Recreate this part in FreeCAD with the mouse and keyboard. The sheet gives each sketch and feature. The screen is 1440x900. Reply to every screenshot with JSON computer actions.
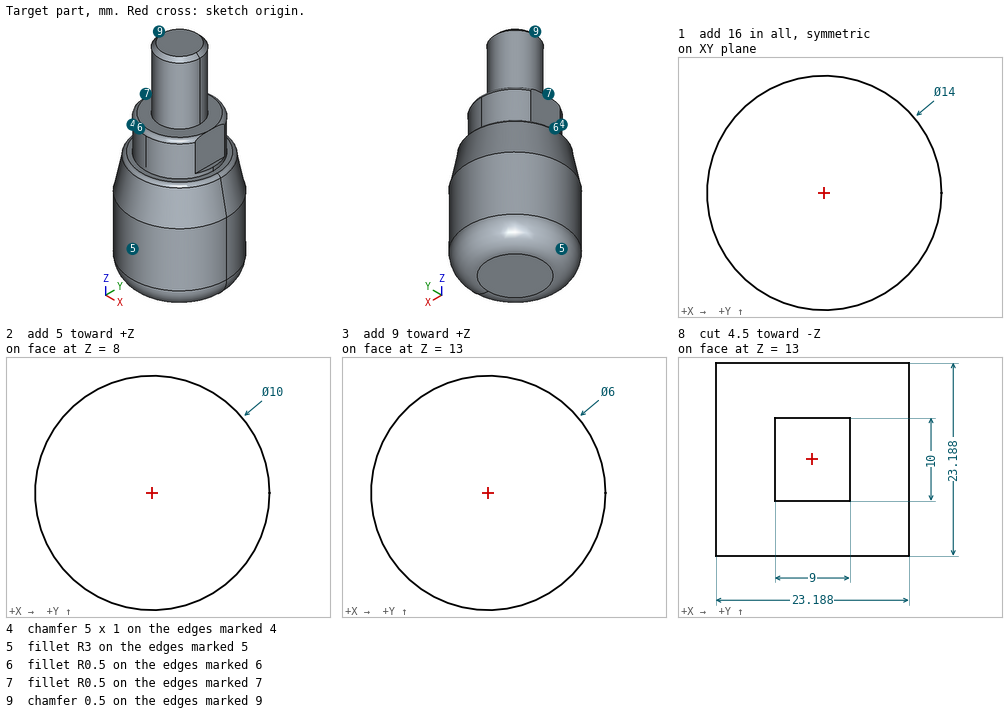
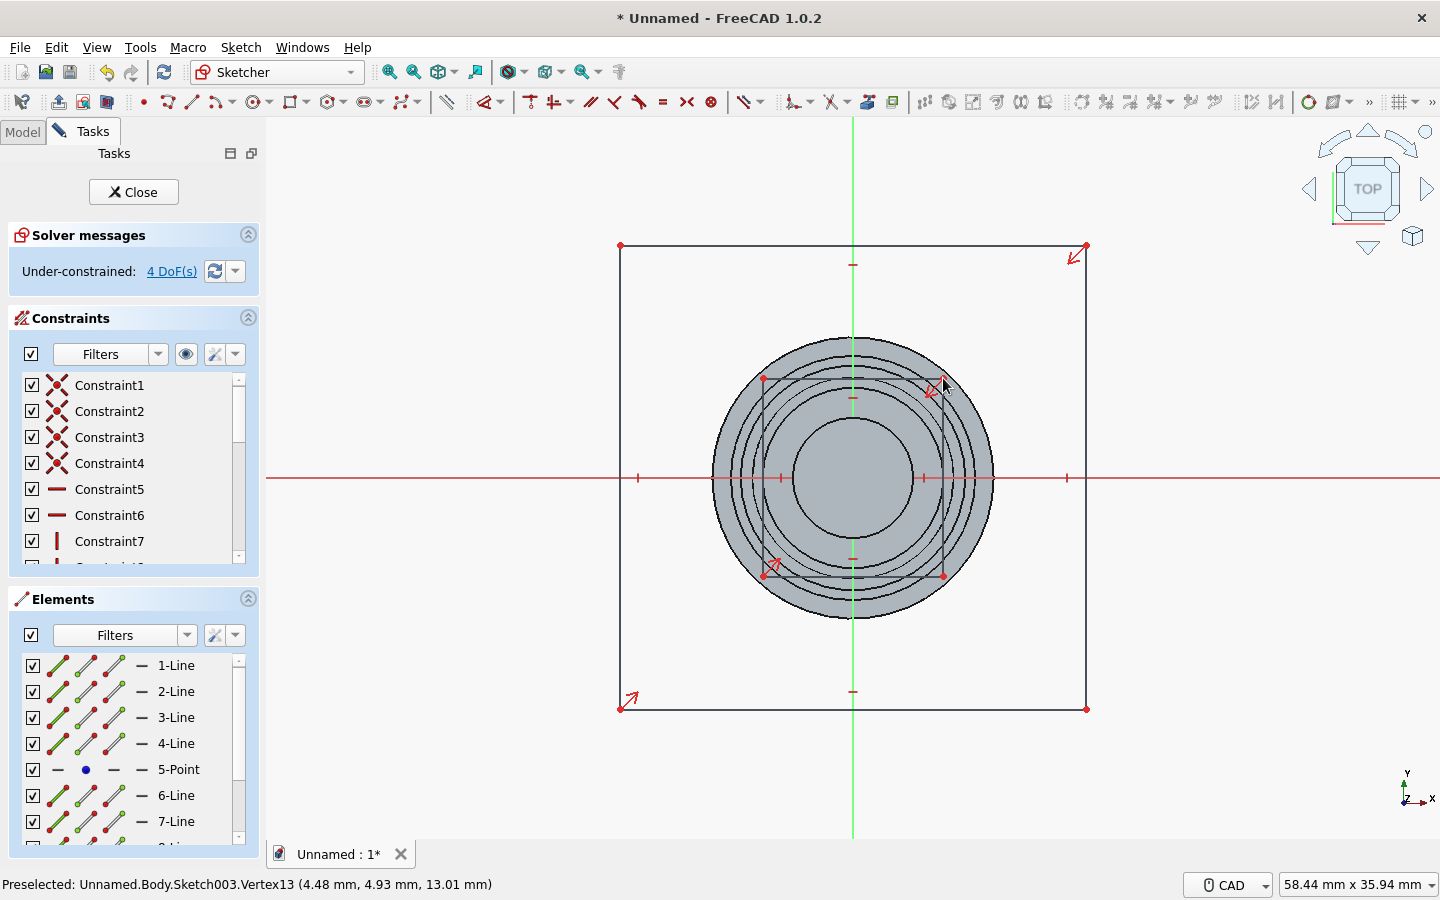
{"action": "left_click", "coordinate": [817, 577]}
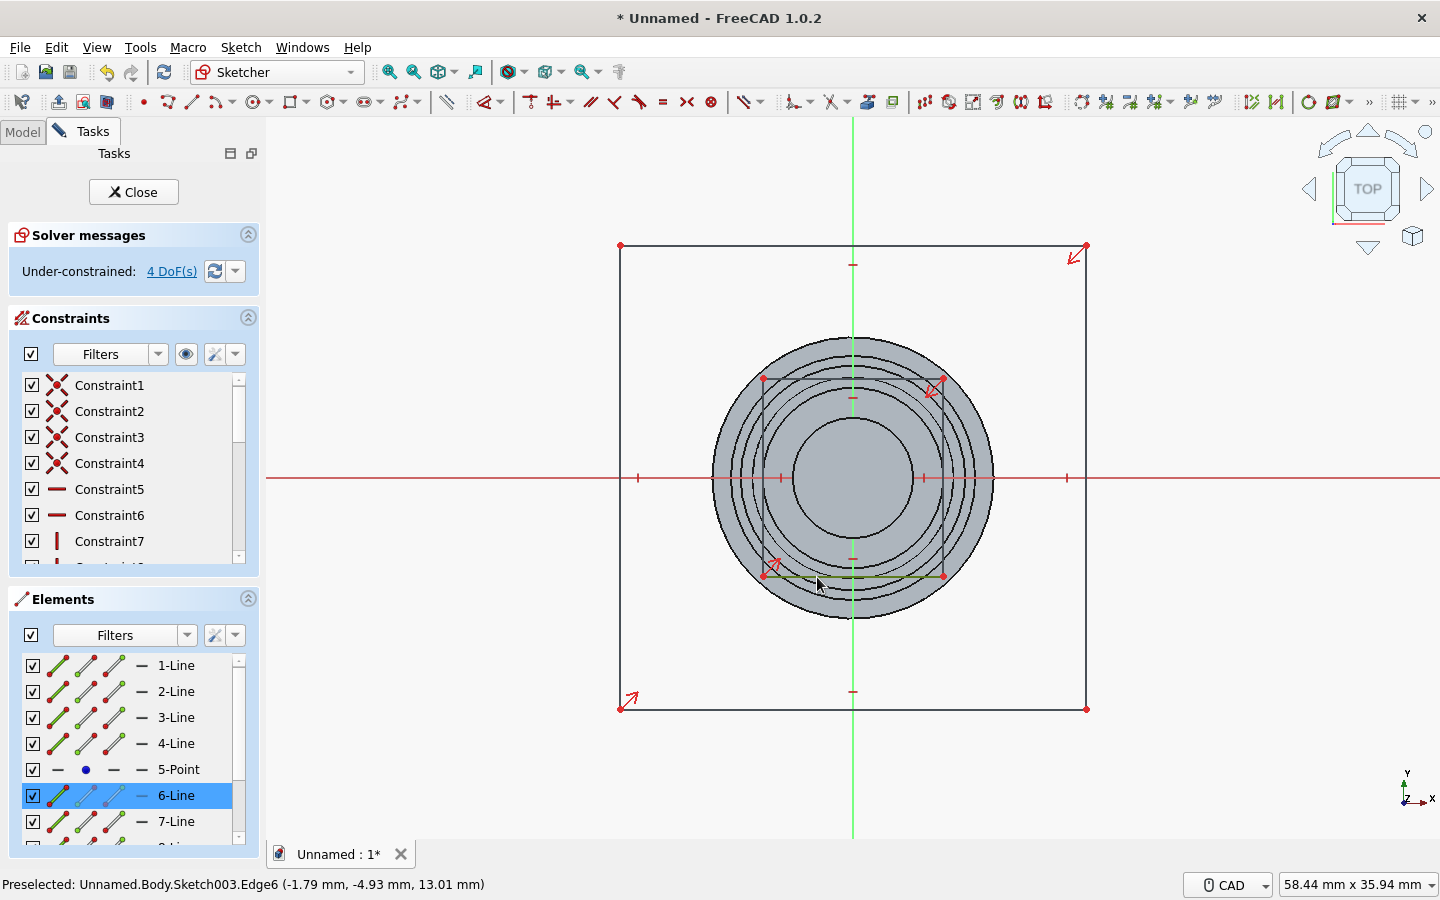
{"action": "key", "text": "l"}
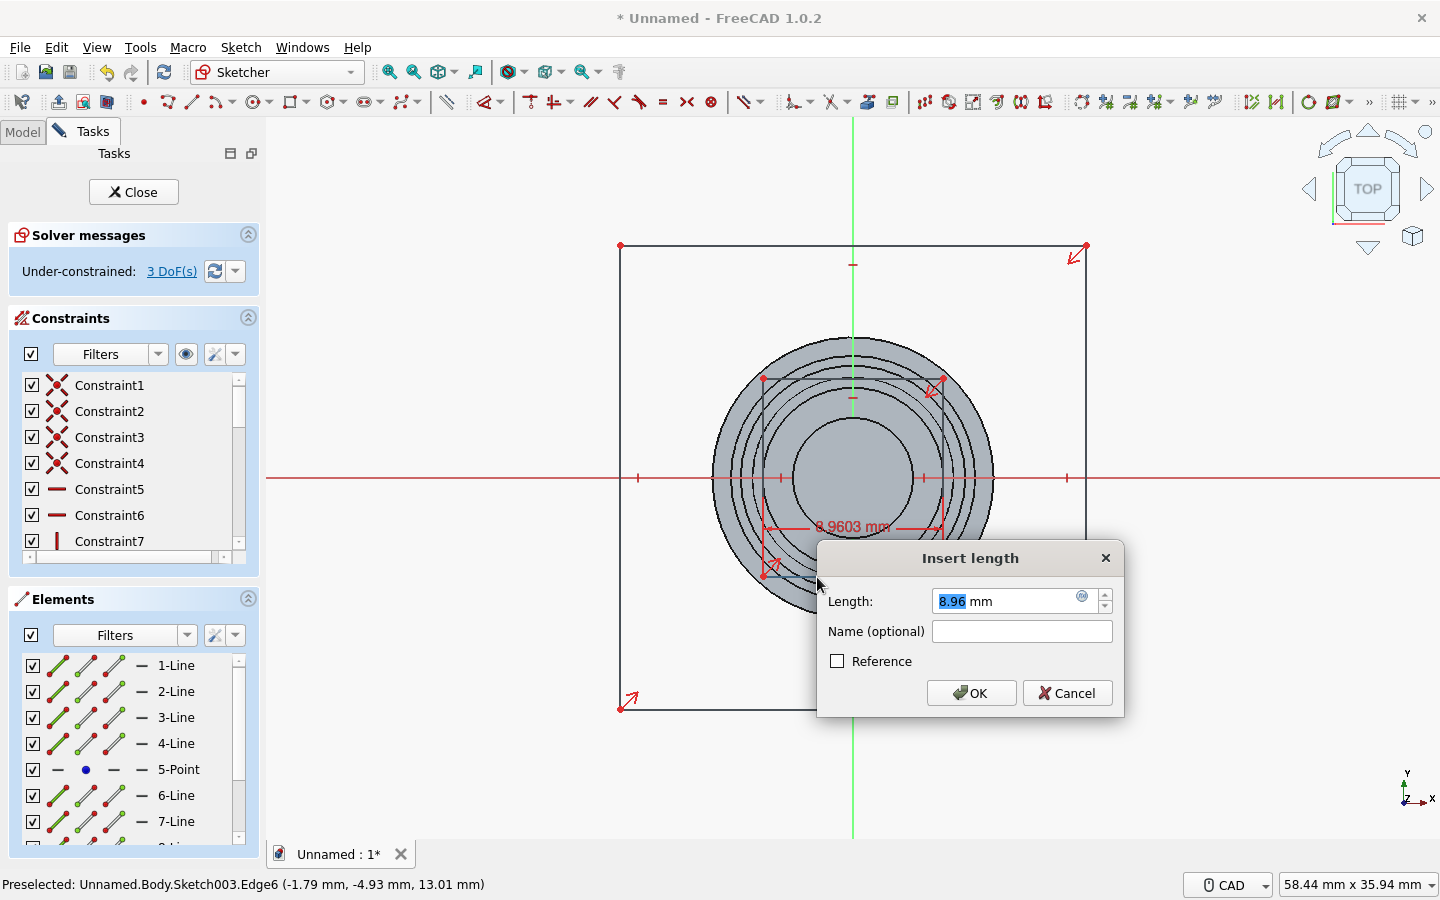
{"action": "type", "text": "9"}
{"action": "key", "text": "Return"}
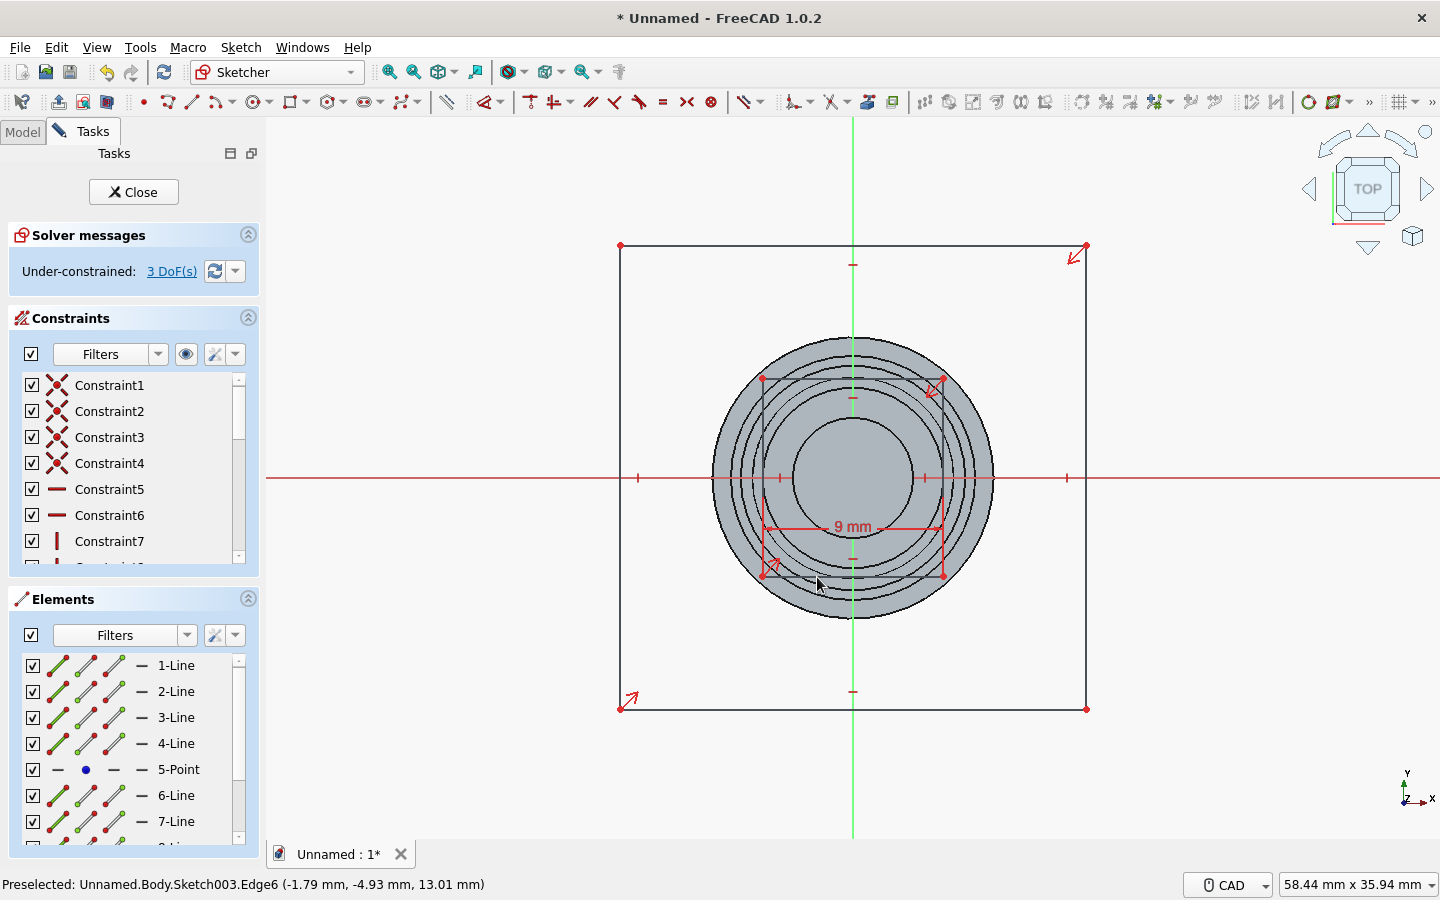
{"action": "left_click", "coordinate": [943, 518]}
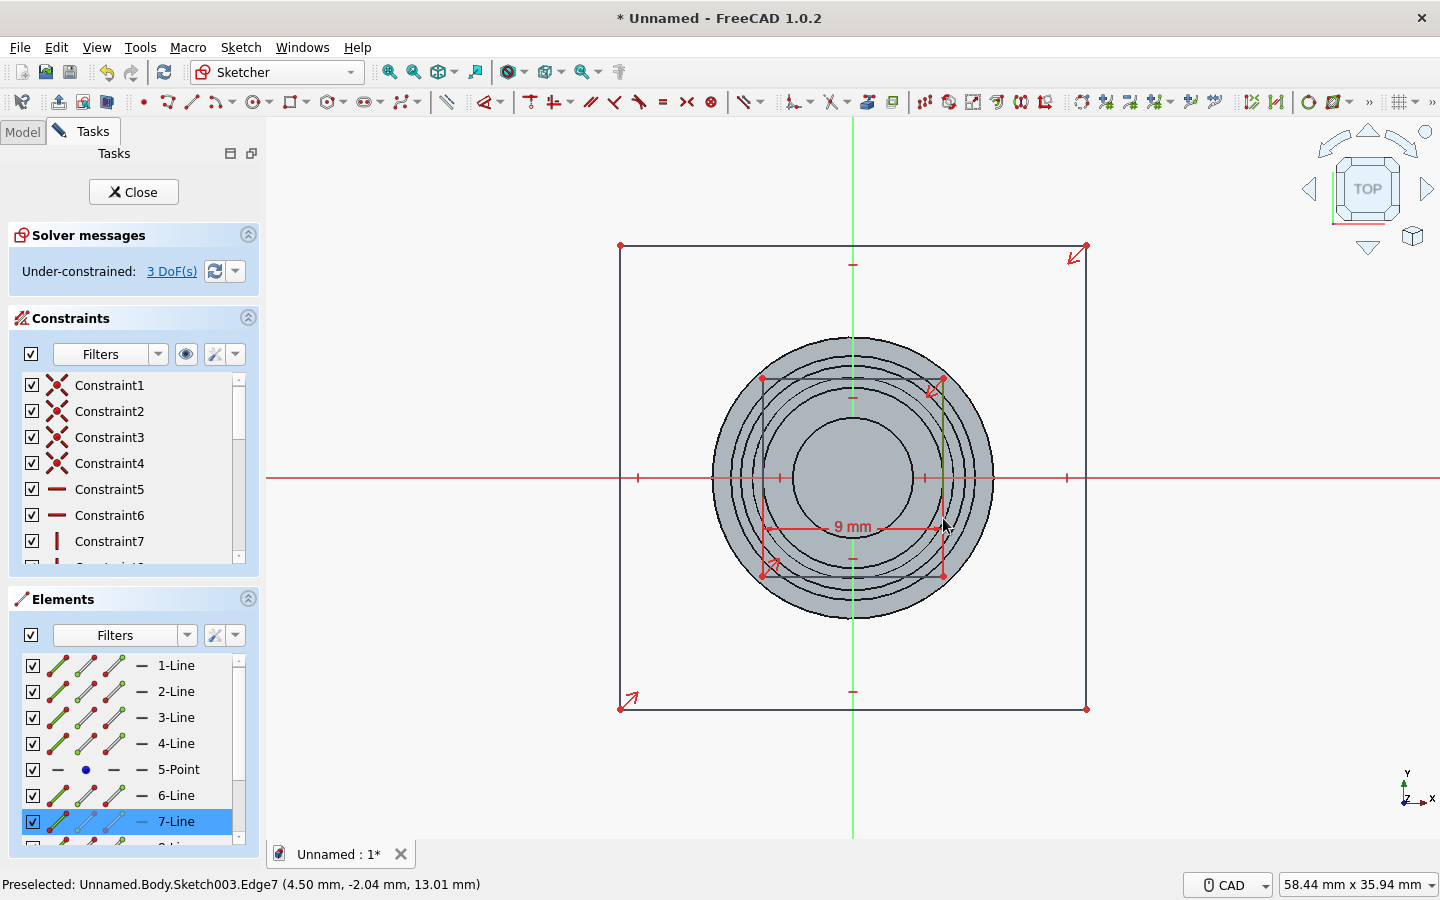
{"action": "left_click", "coordinate": [502, 102]}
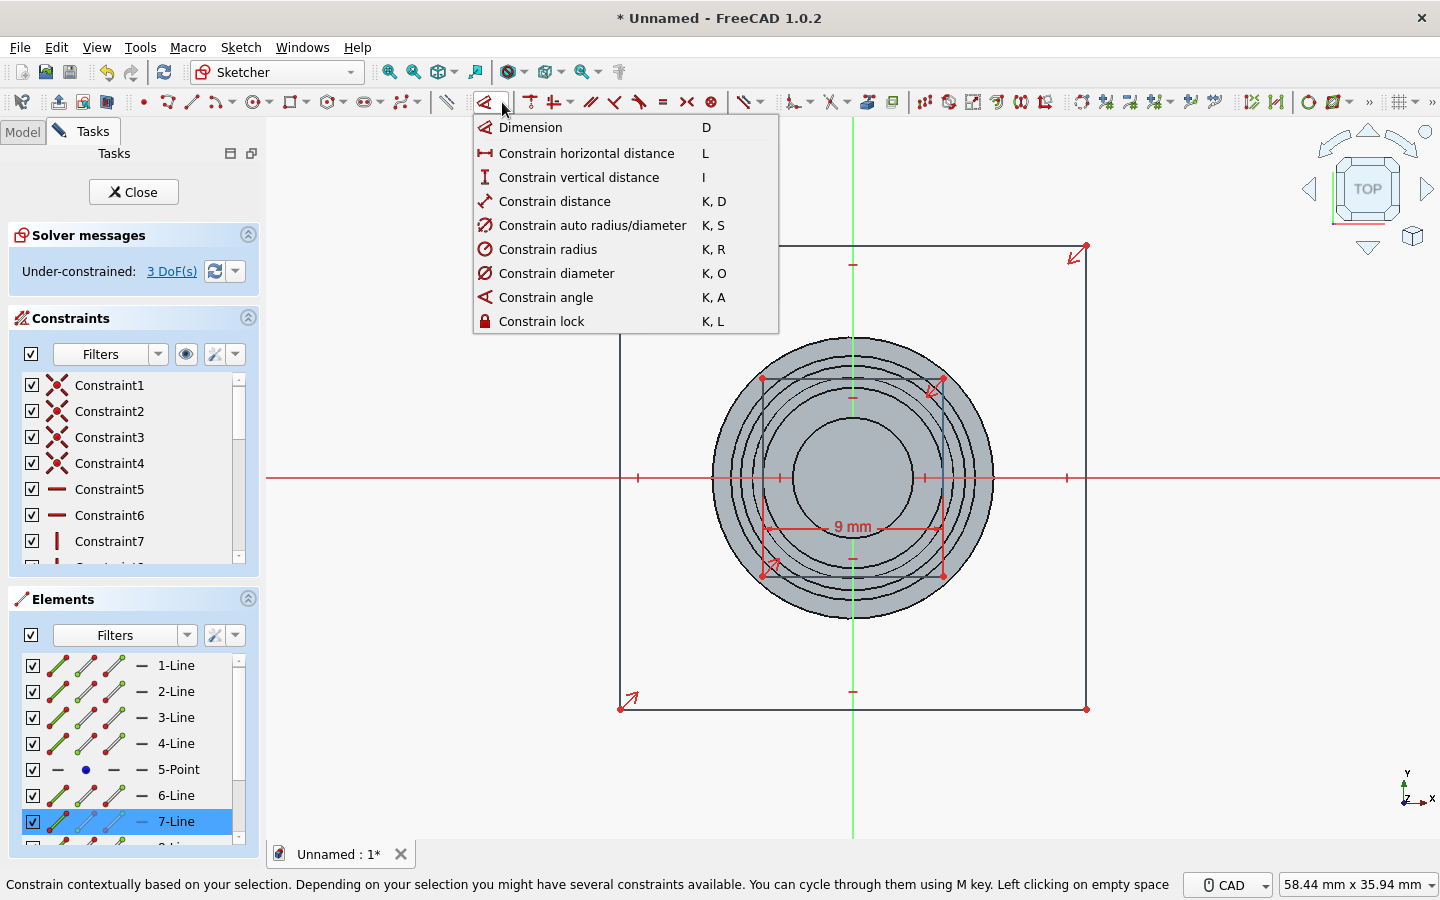
{"action": "left_click", "coordinate": [626, 177]}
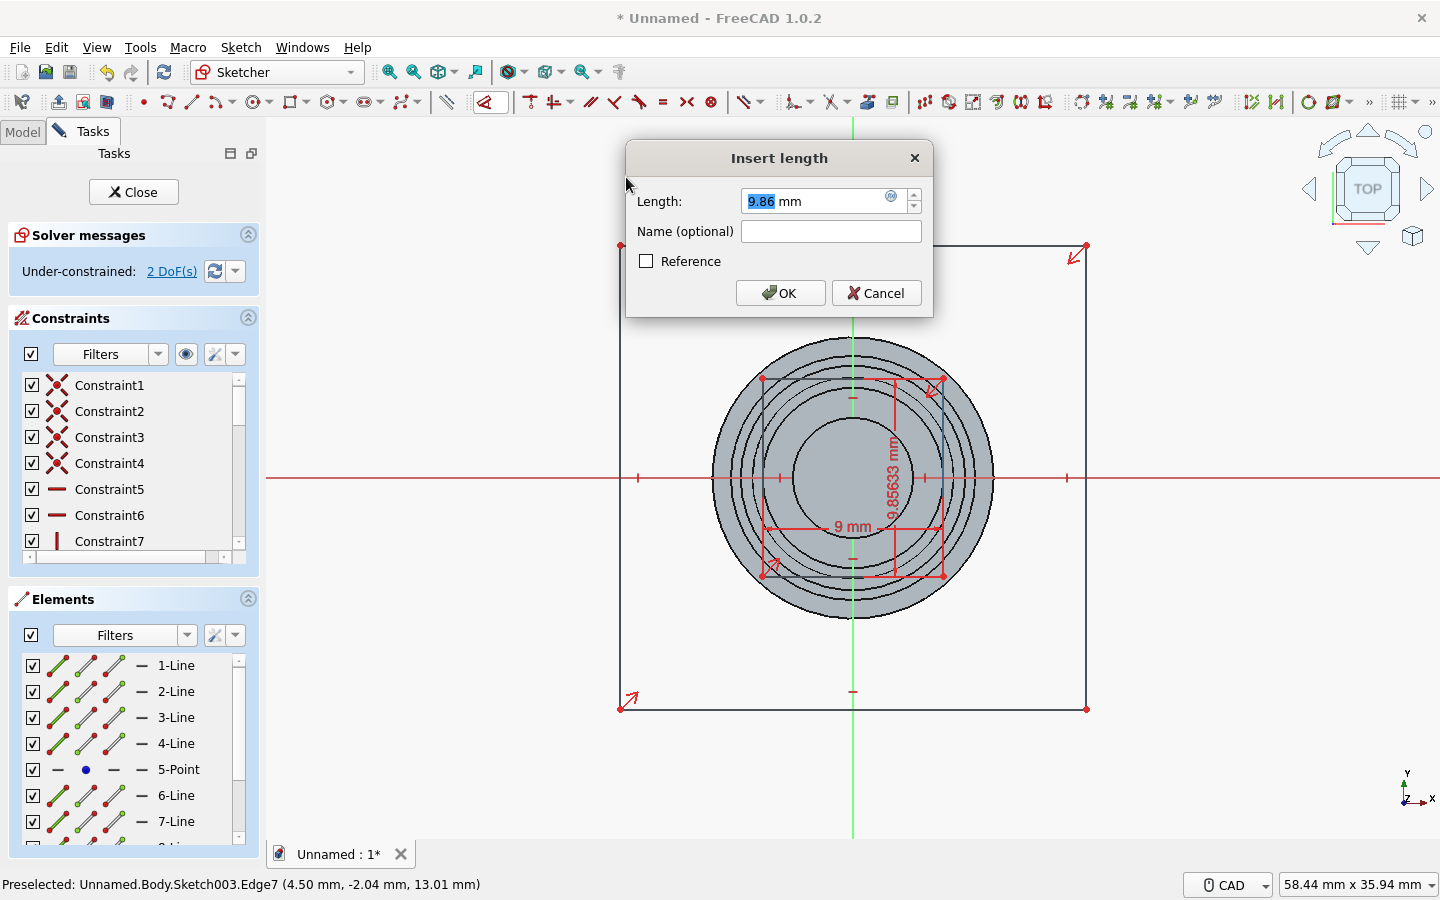
{"action": "type", "text": "10"}
{"action": "key", "text": "Return"}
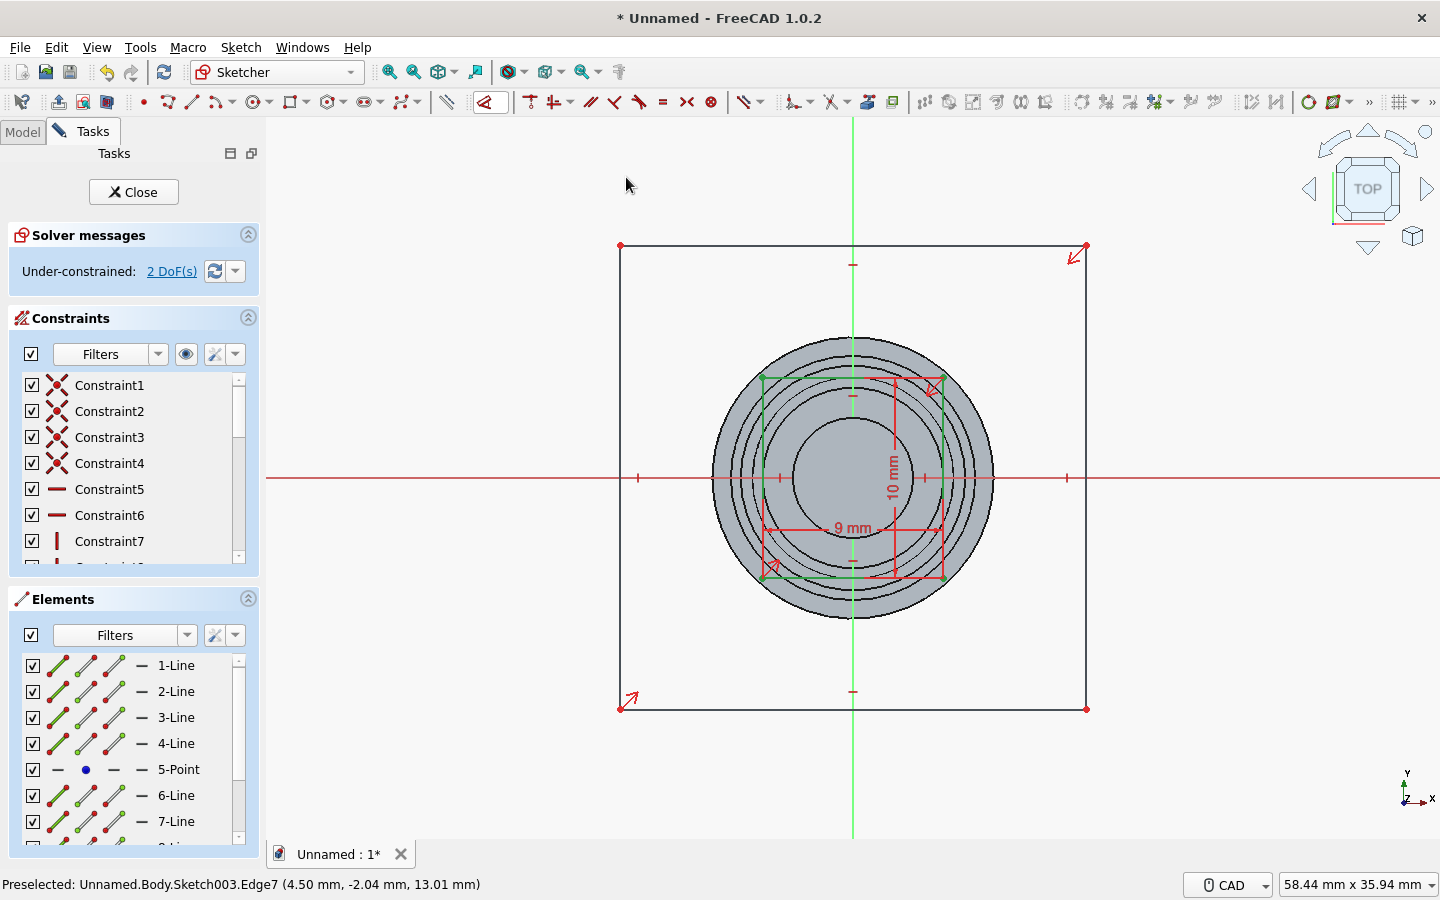
{"action": "left_click", "coordinate": [760, 710]}